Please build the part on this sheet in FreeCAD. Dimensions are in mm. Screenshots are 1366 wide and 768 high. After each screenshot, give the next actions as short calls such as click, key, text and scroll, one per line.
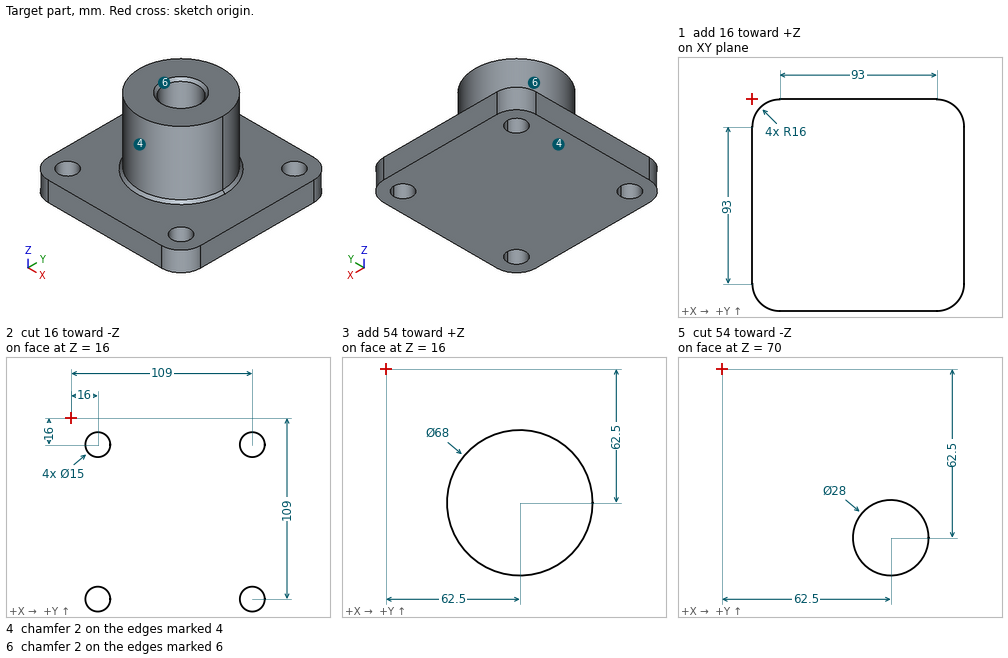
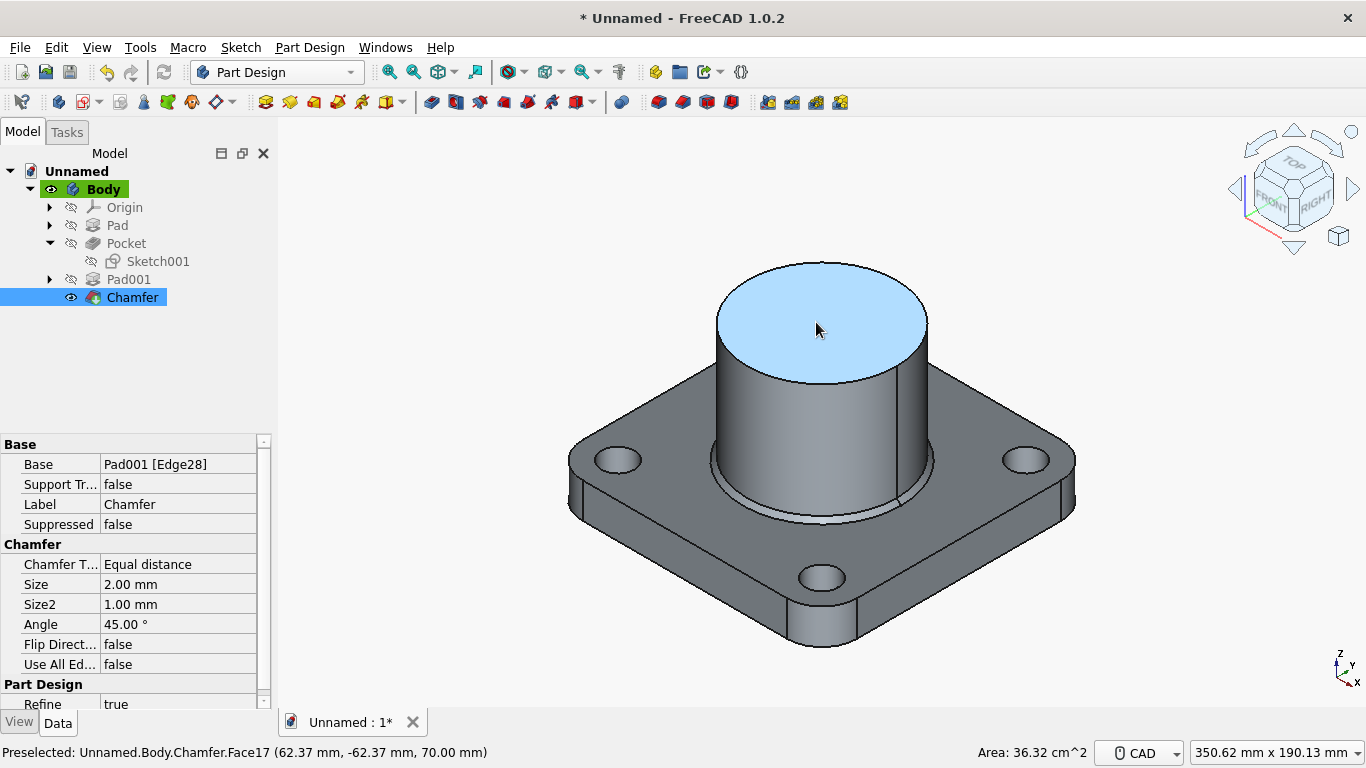
click(84, 102)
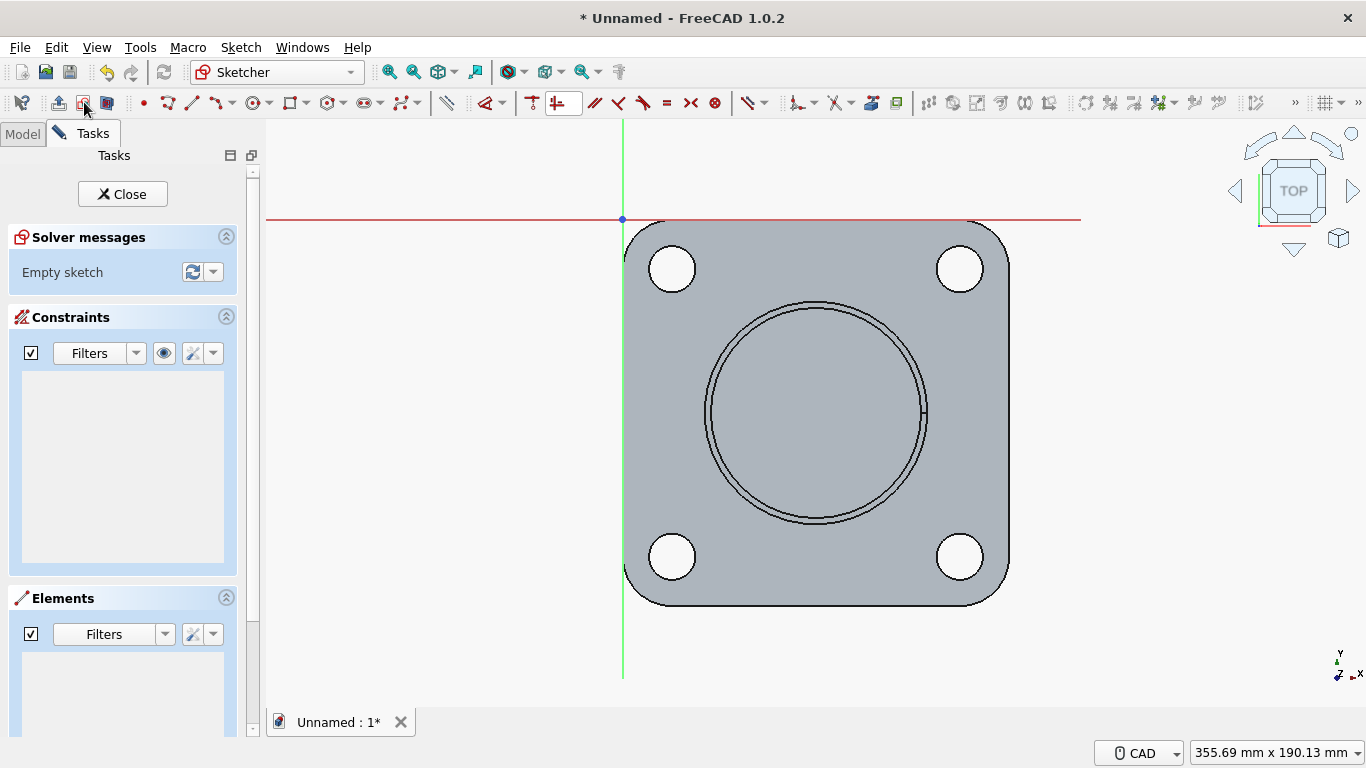
scroll(838, 413, up, 7)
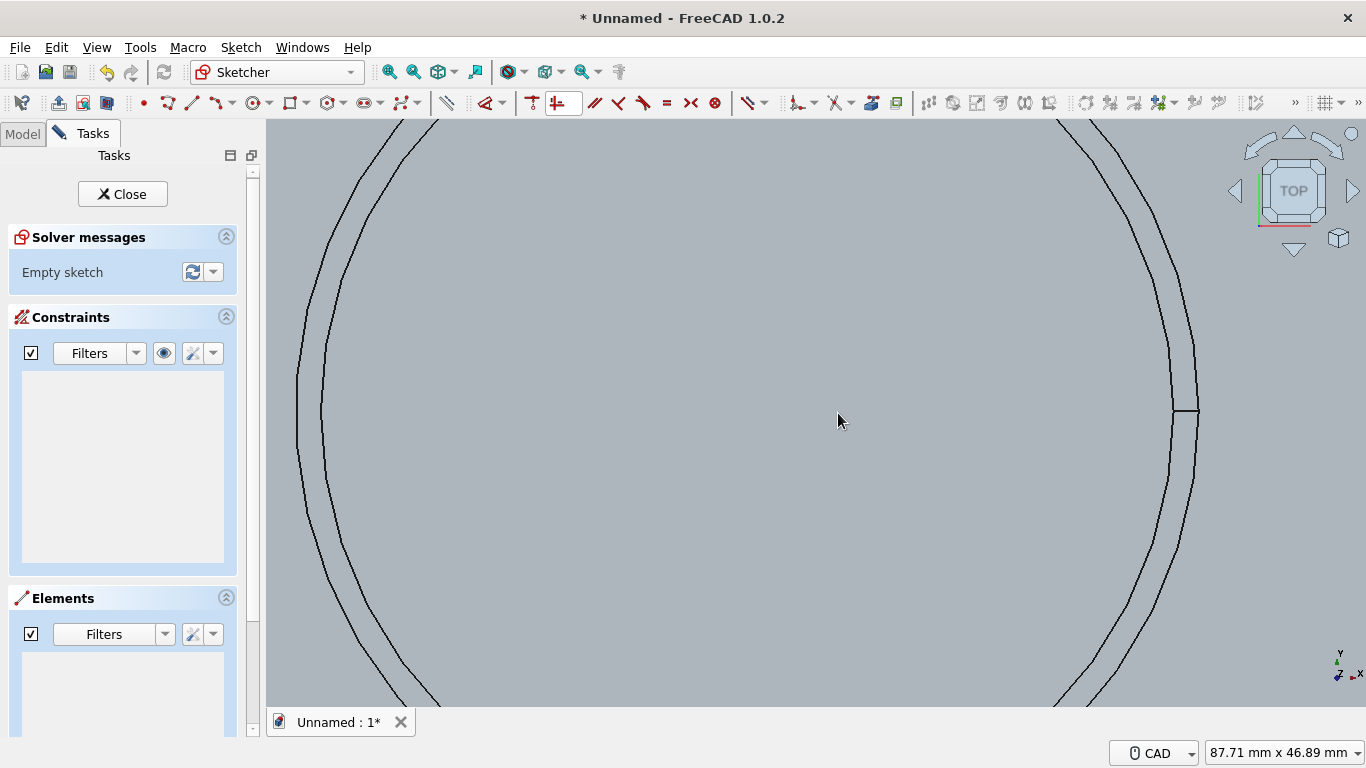
key(g)
key(c)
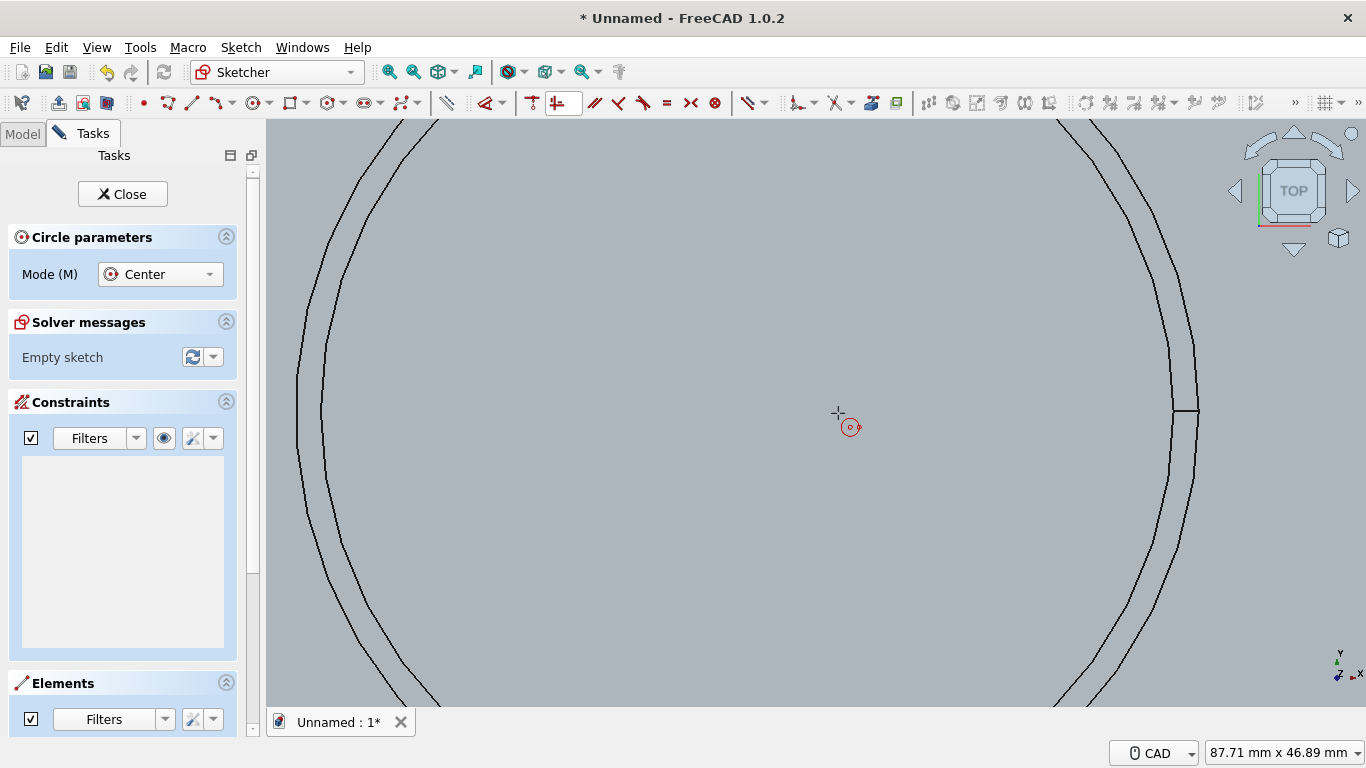
click(747, 411)
move(871, 287)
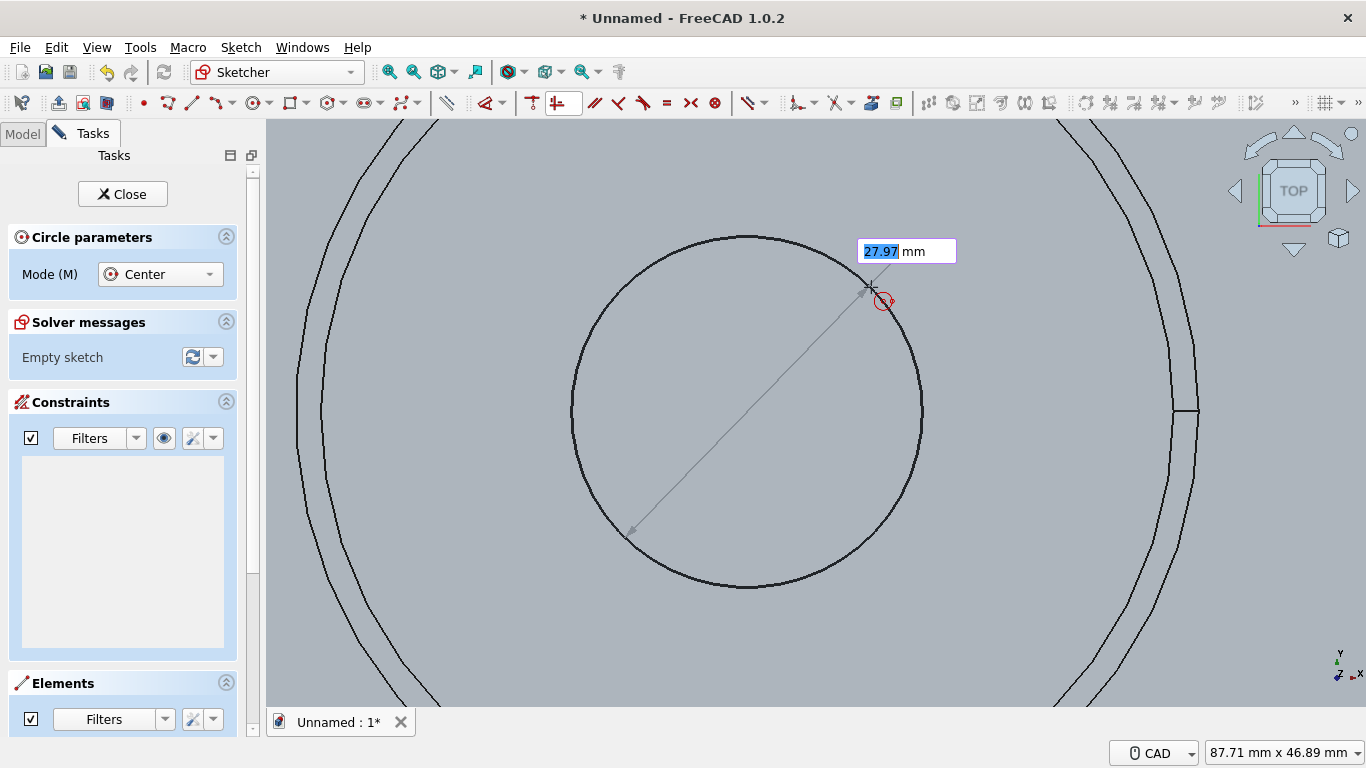
text(28)
key(Return)
key(Escape)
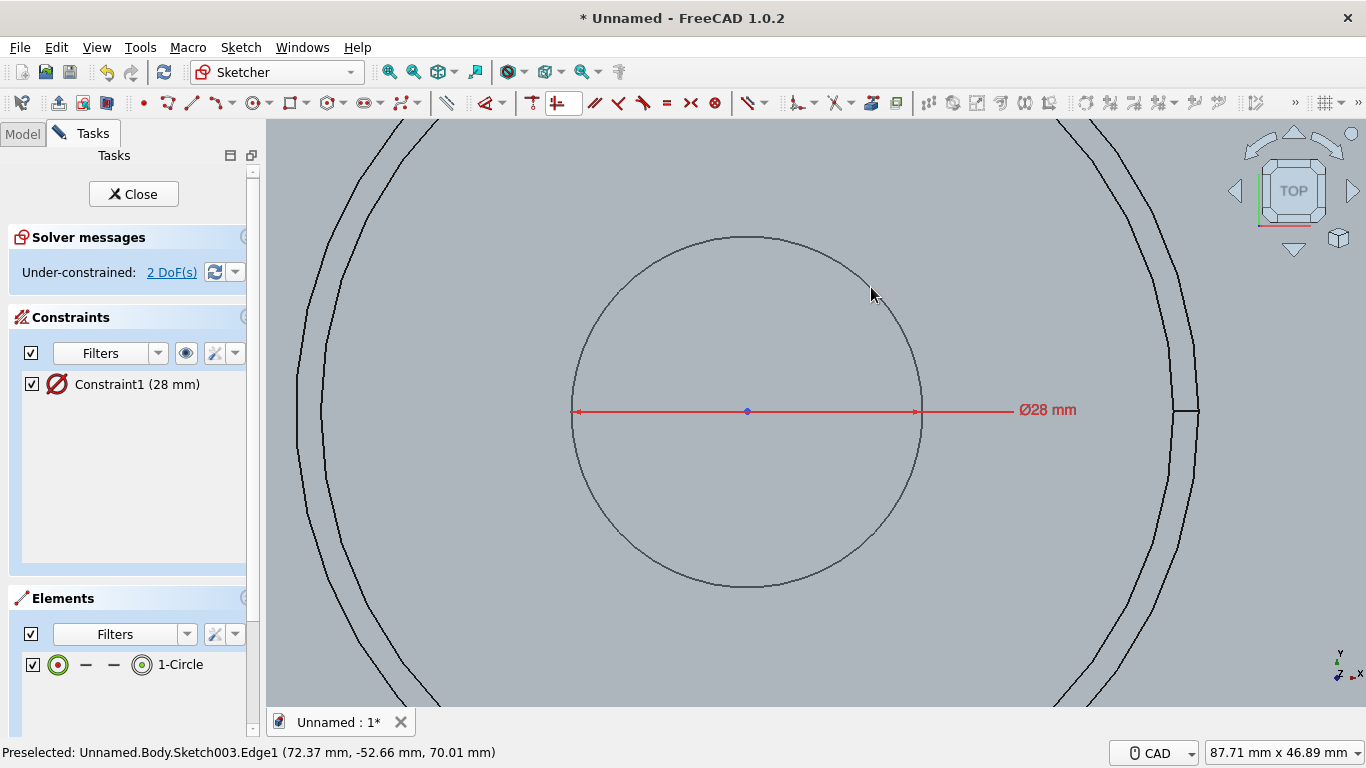
key(d)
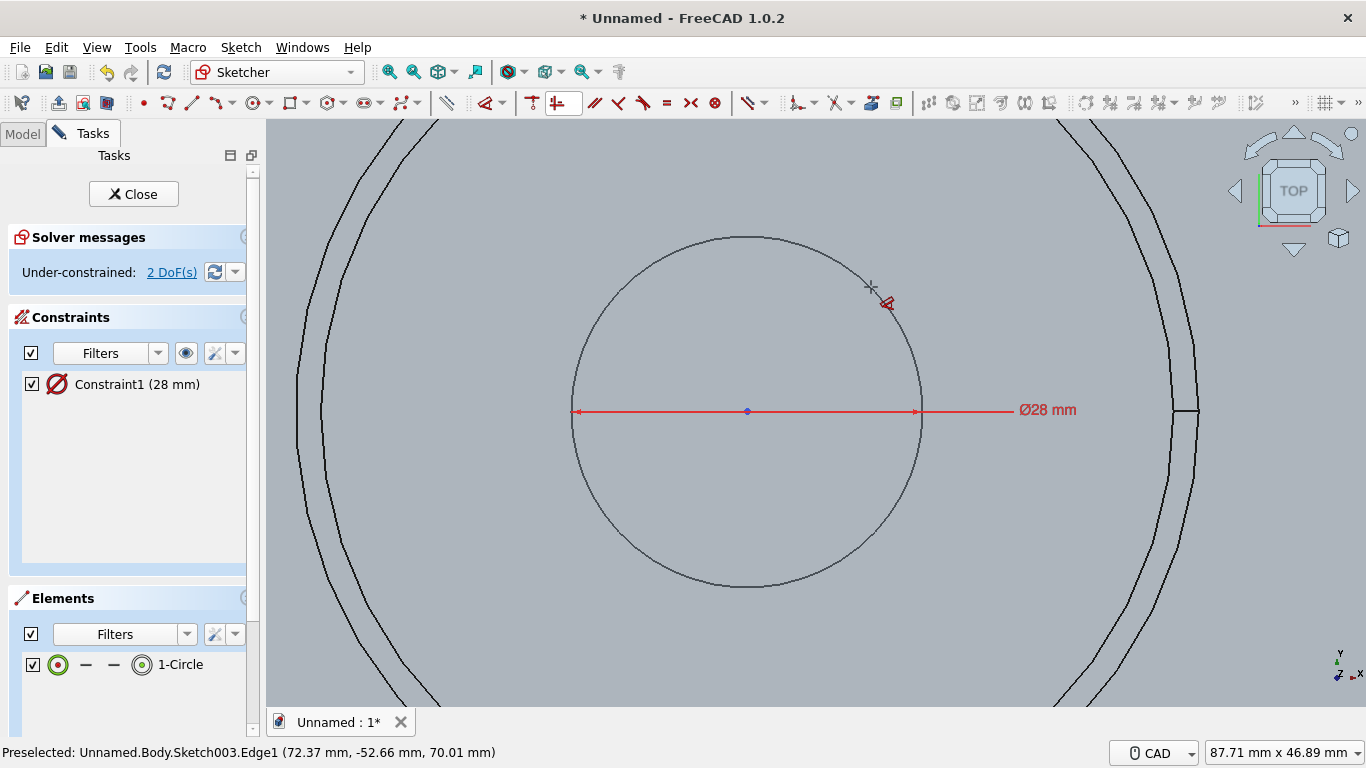
click(747, 412)
click(521, 446)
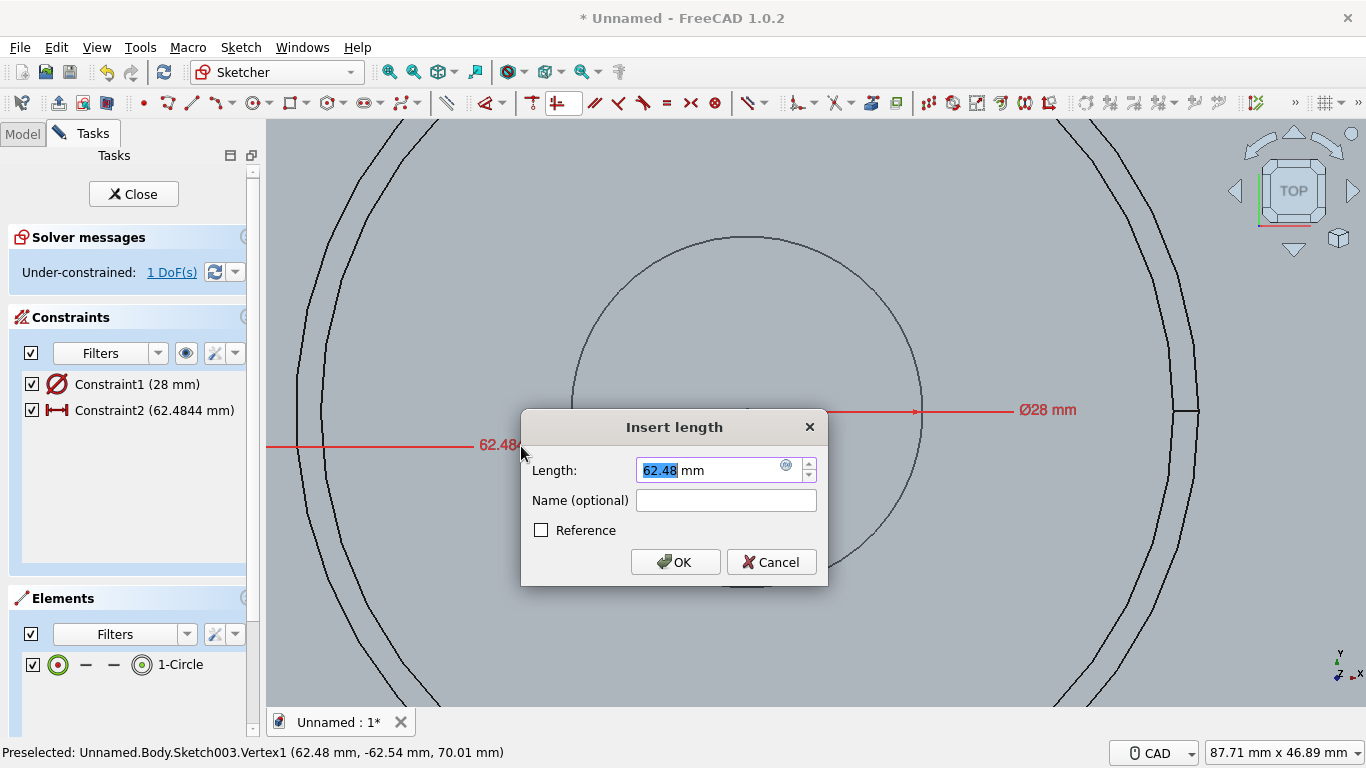
text(62.5)
key(Return)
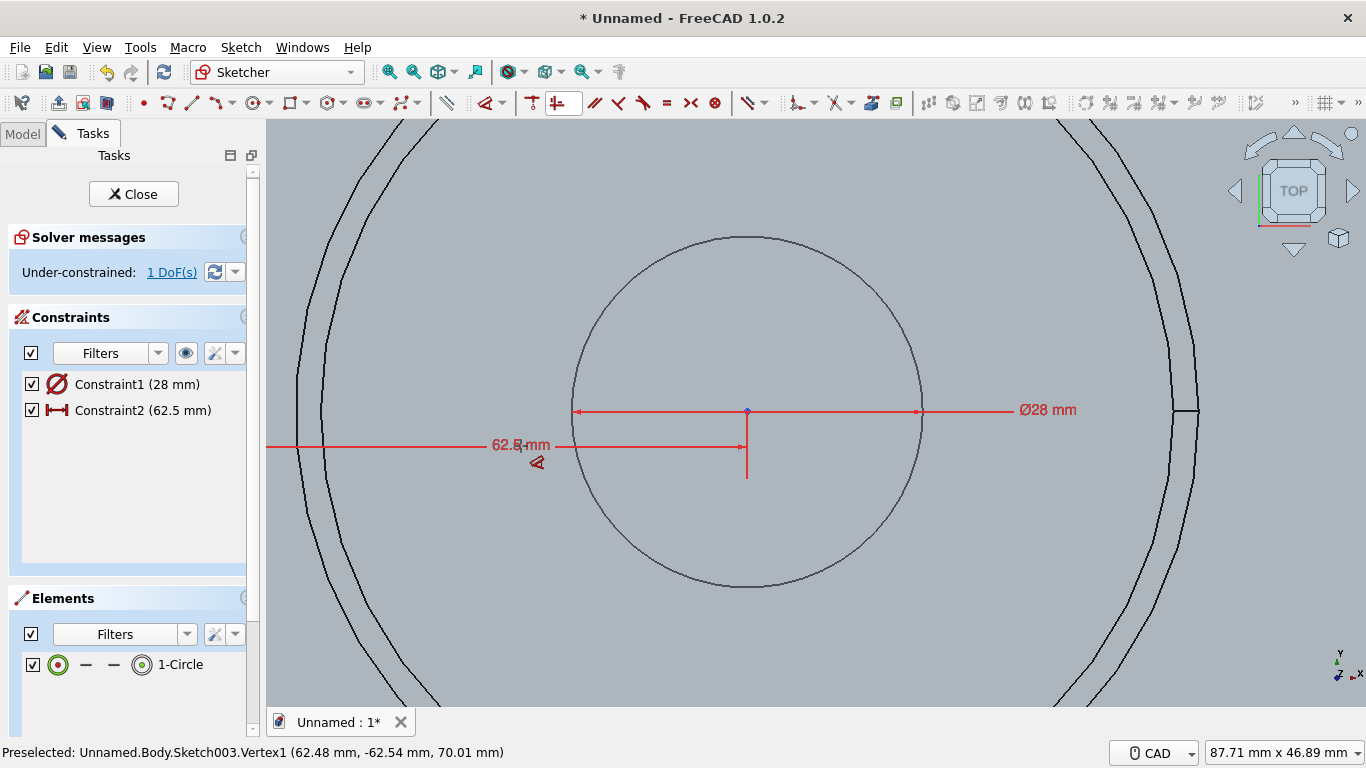
click(747, 412)
click(781, 279)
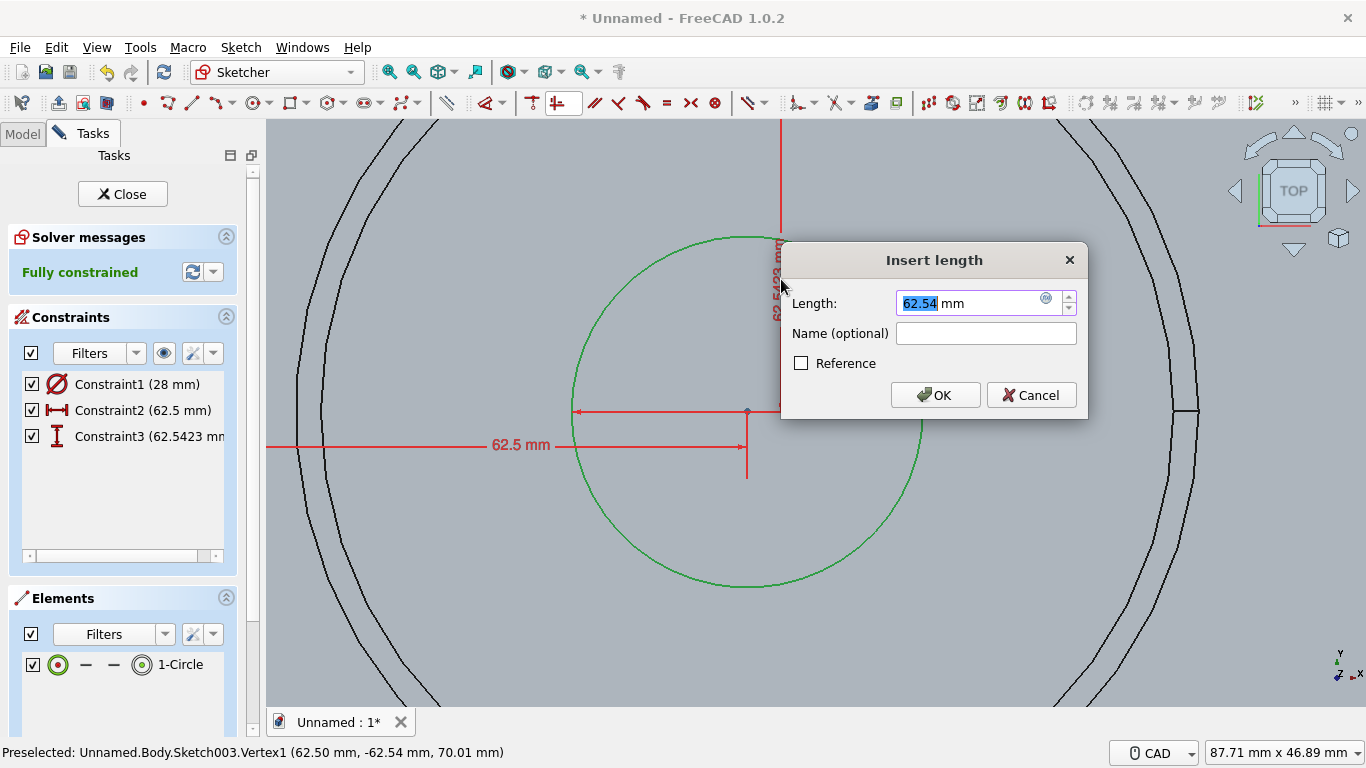
text(62.5)
key(Return)
key(Escape)